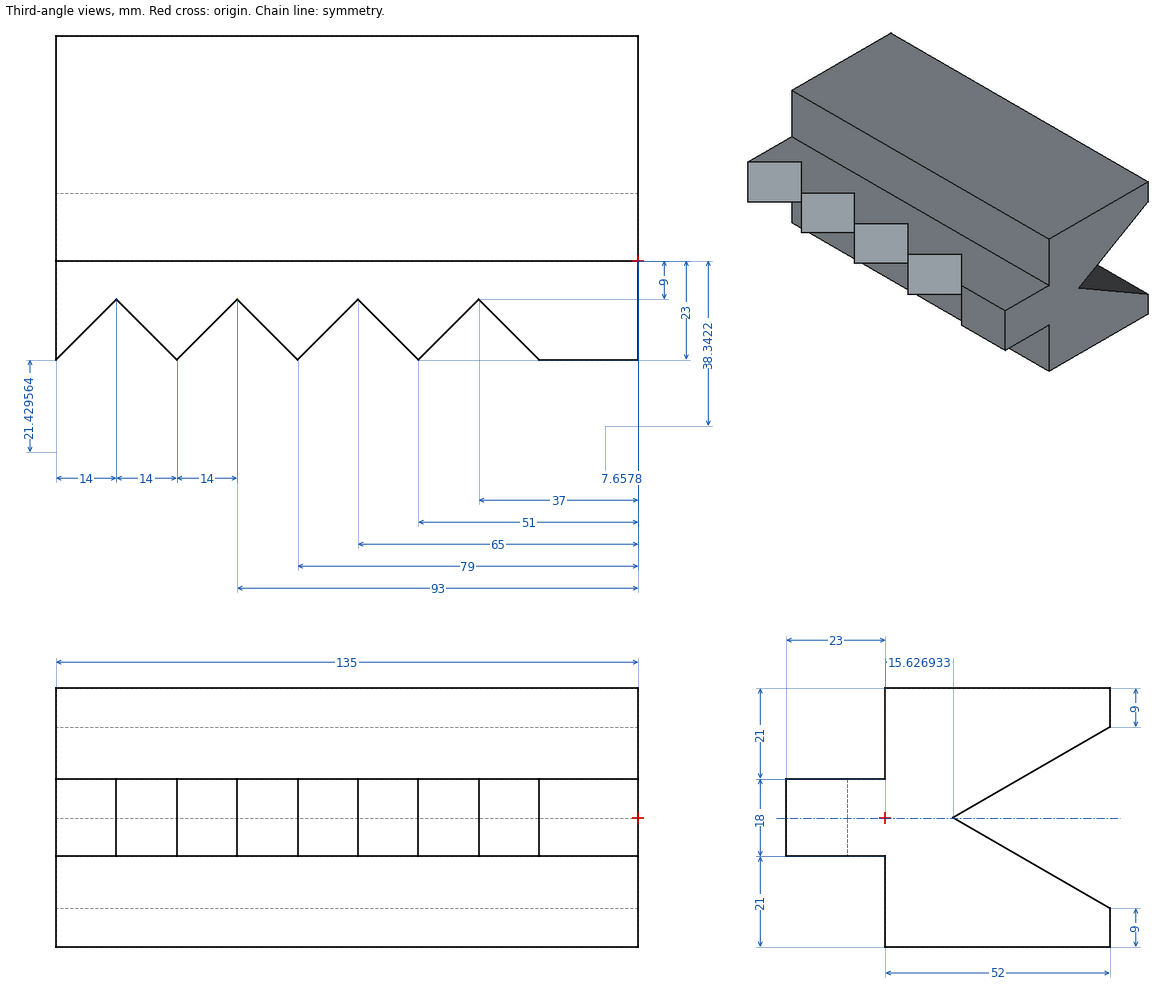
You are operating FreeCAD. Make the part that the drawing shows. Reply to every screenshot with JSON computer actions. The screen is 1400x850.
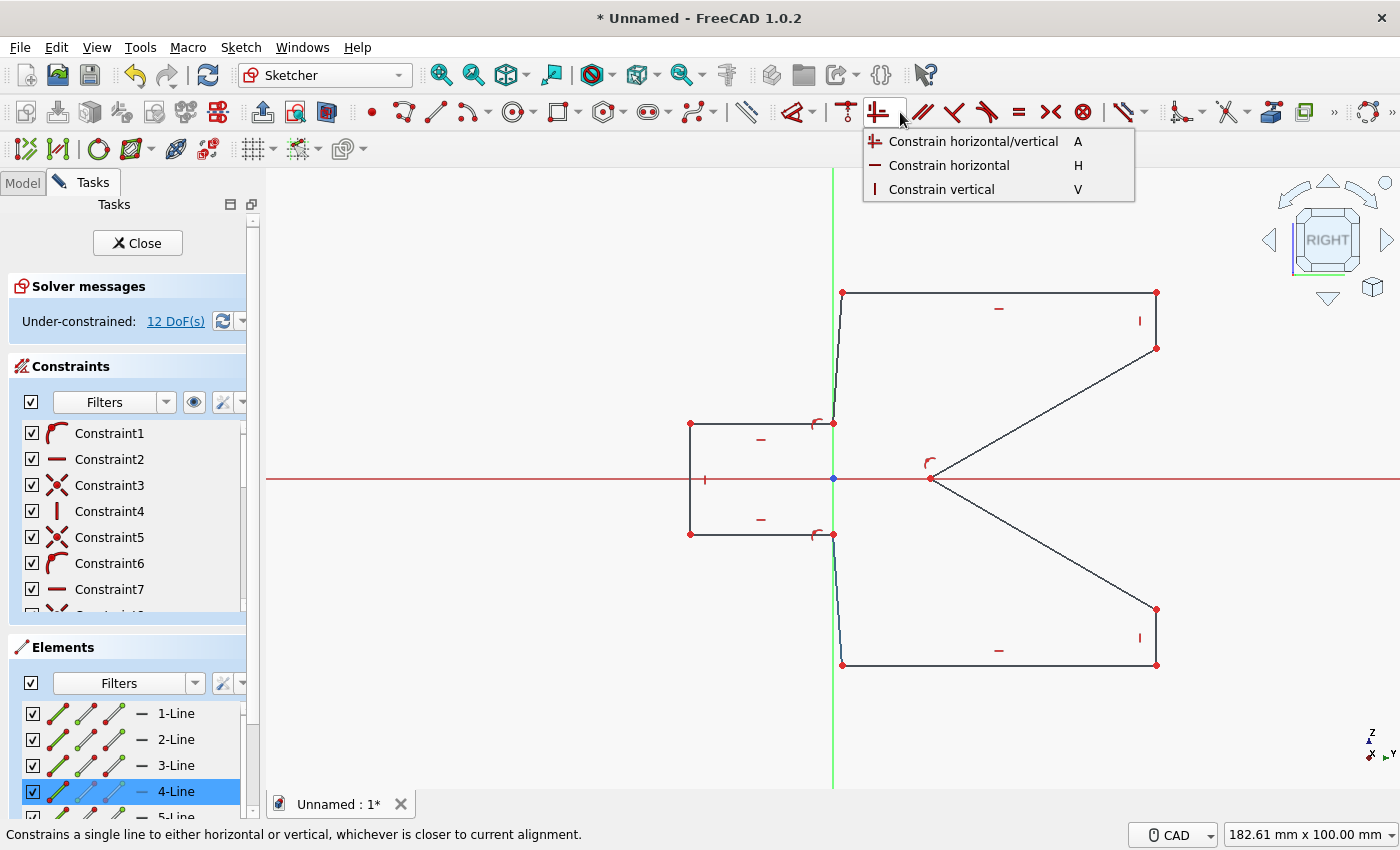
{"action": "left_click", "coordinate": [999, 189]}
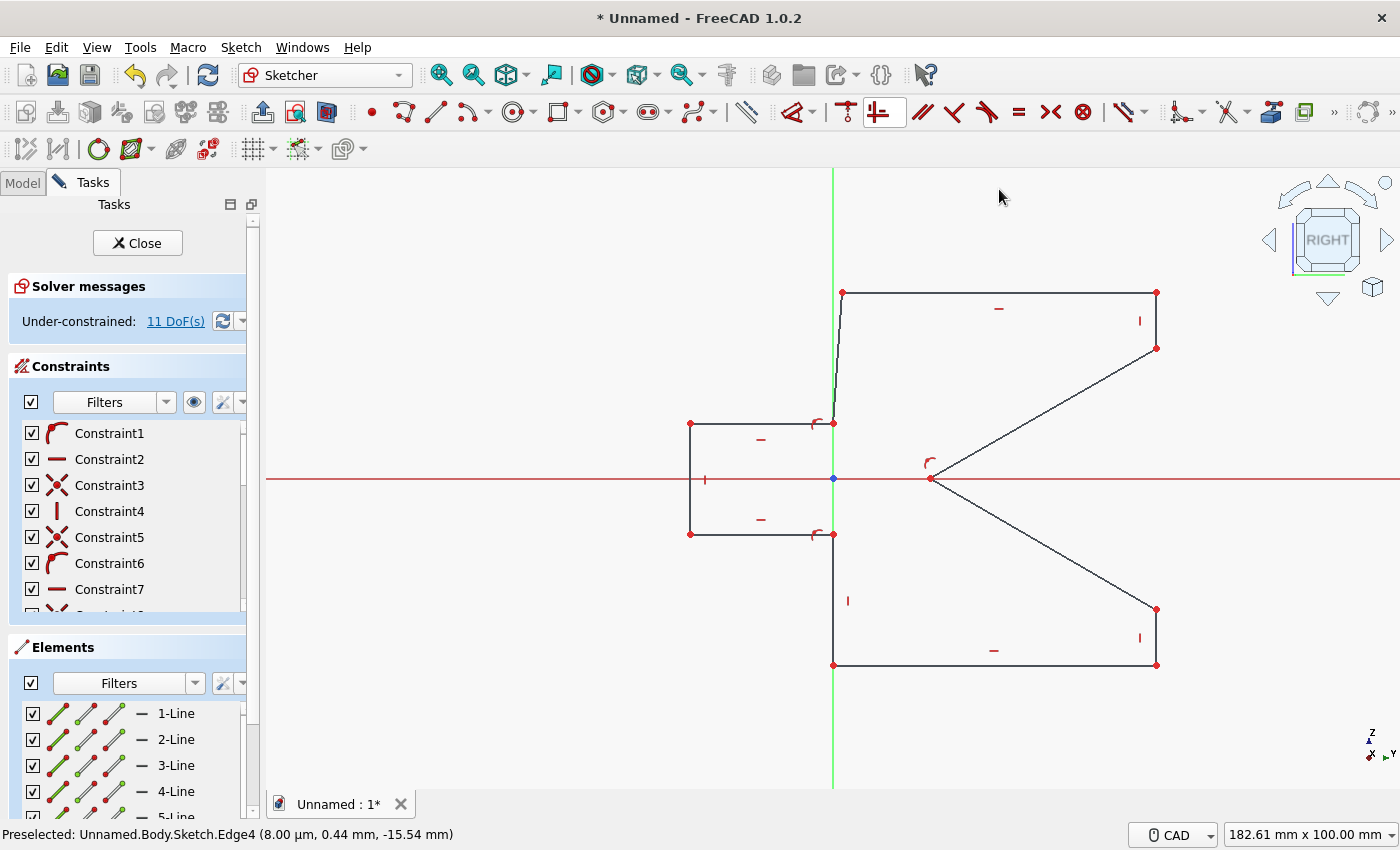
{"action": "left_click", "coordinate": [836, 385]}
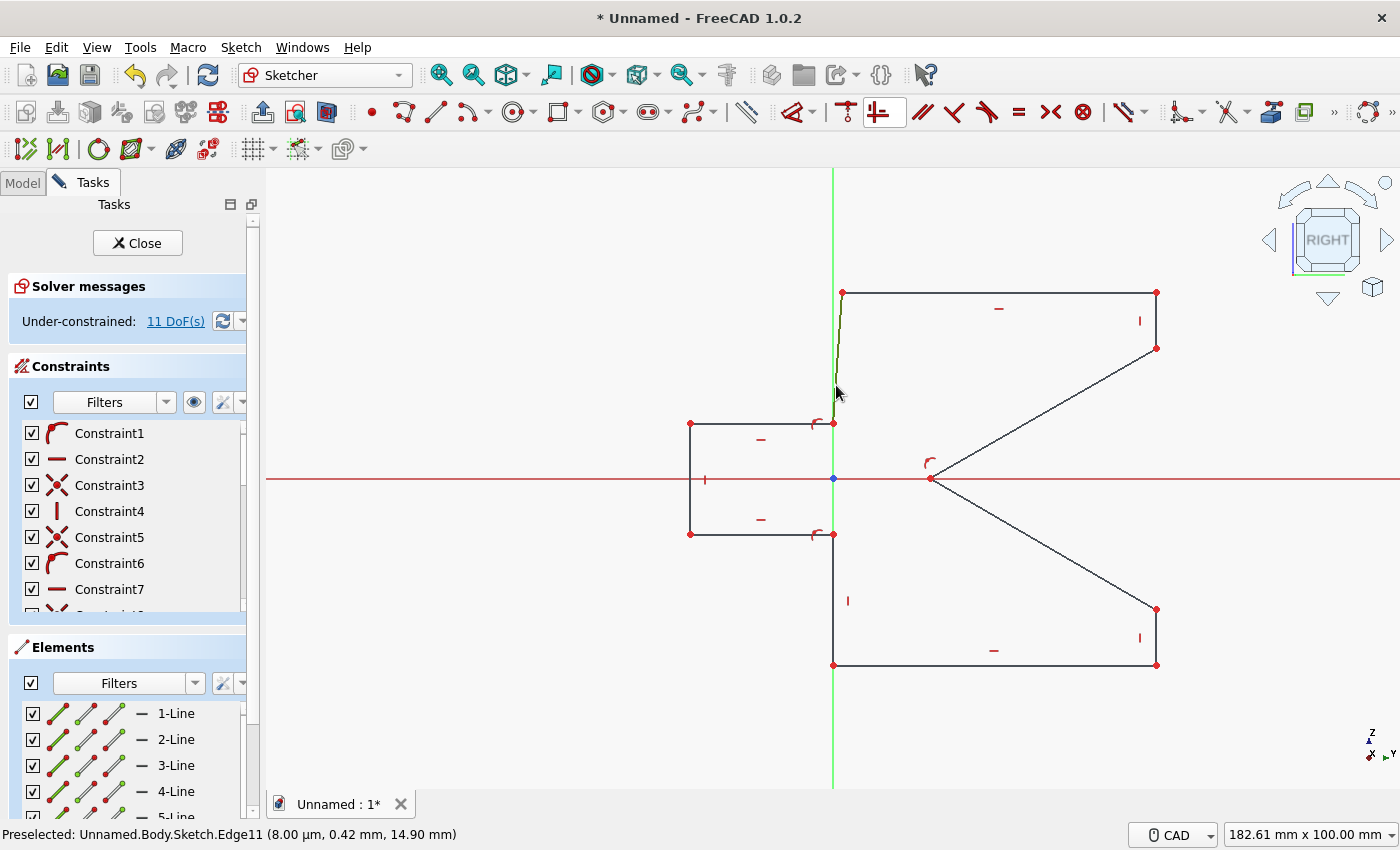
{"action": "key", "text": "v"}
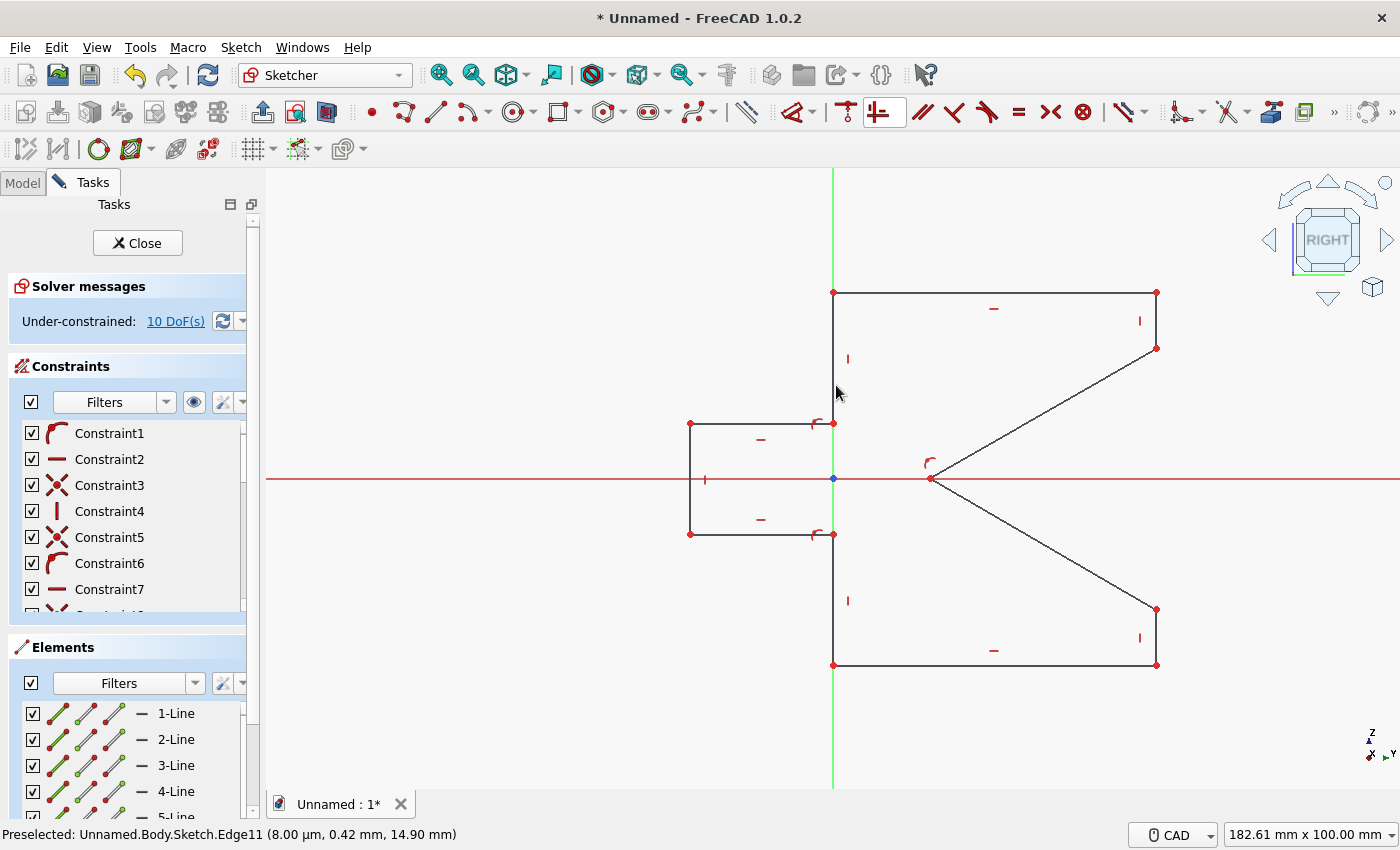
{"action": "left_click", "coordinate": [1156, 610]}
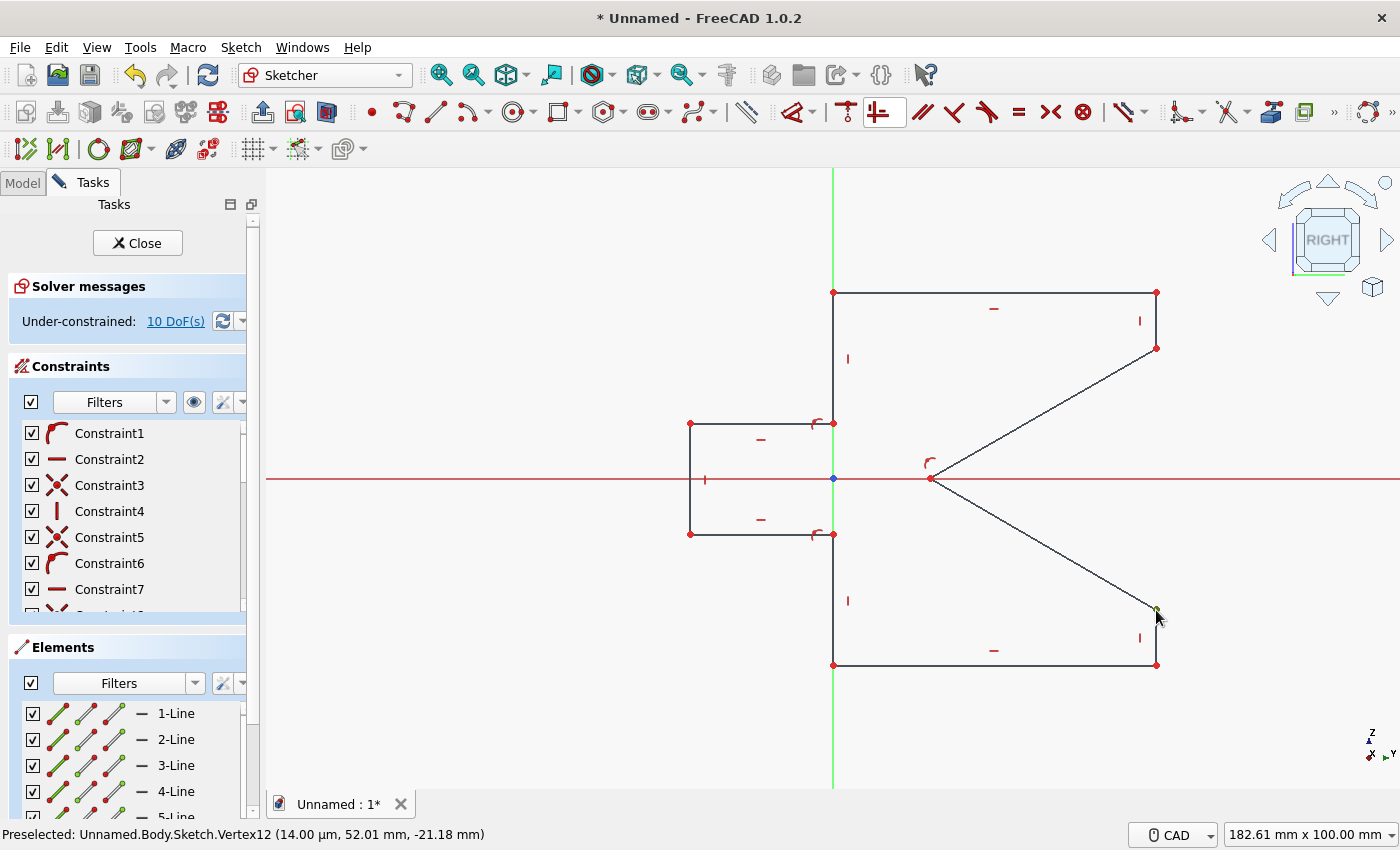
{"action": "left_click", "coordinate": [1156, 349]}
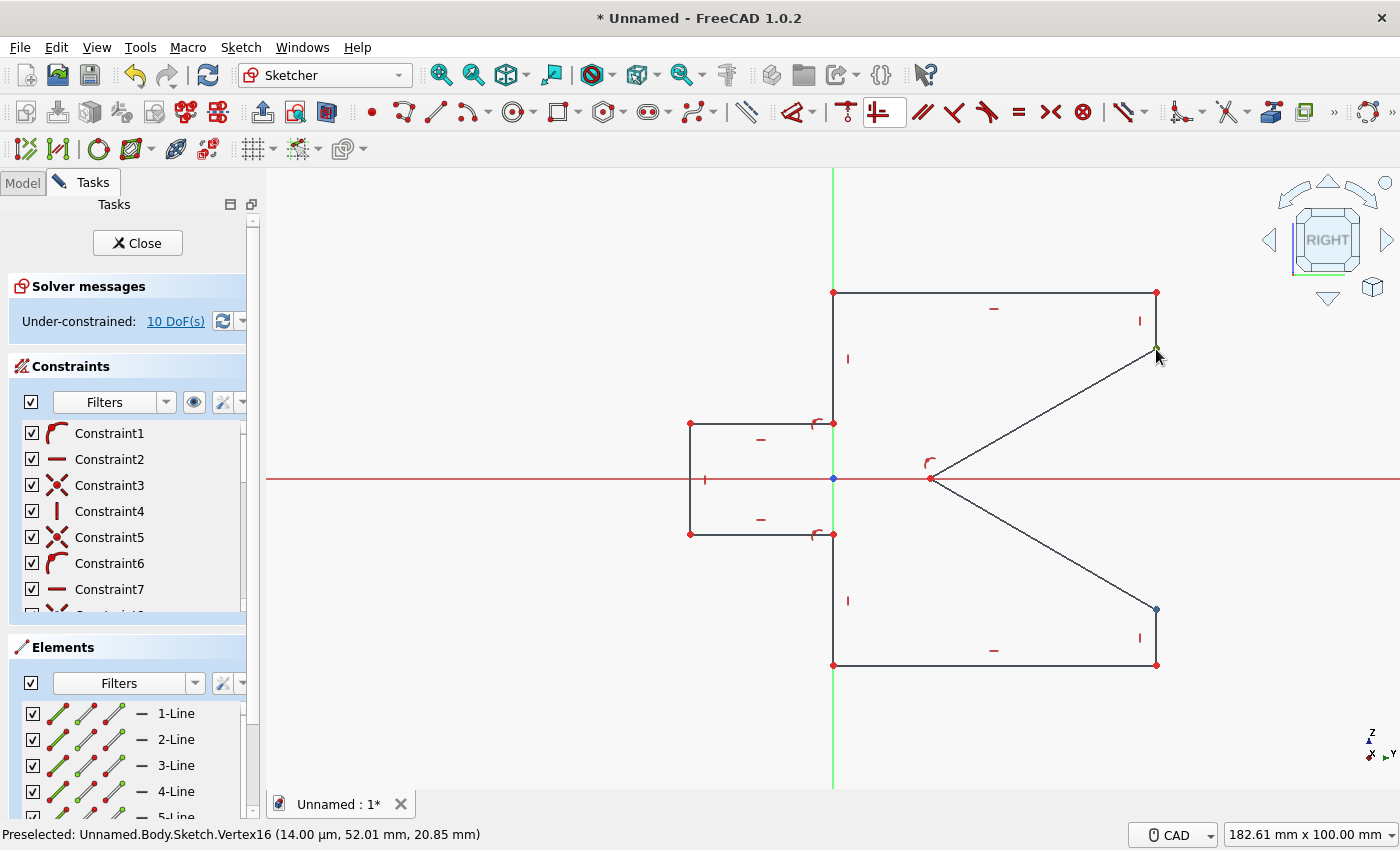
{"action": "left_click", "coordinate": [361, 478]}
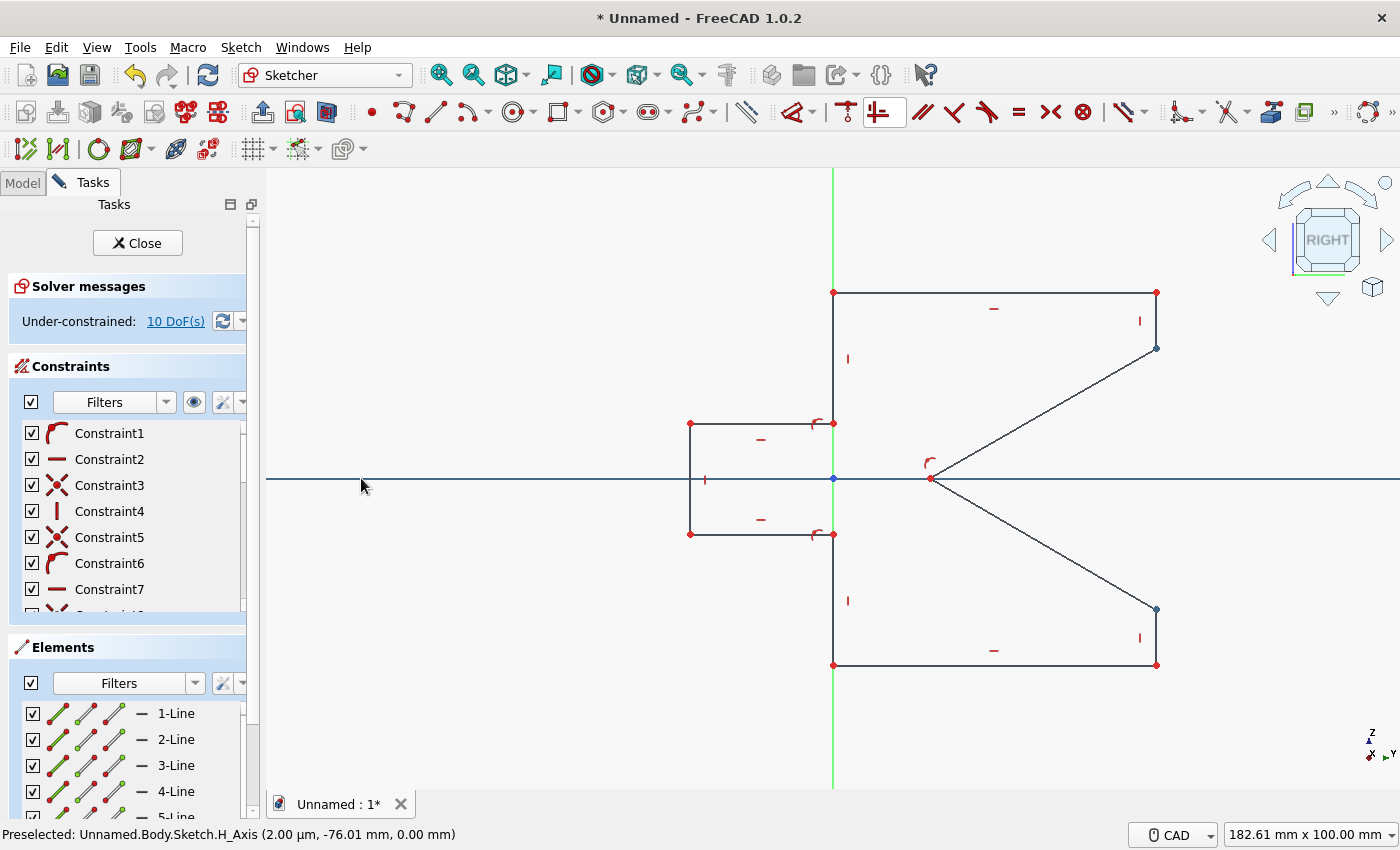
{"action": "left_click", "coordinate": [1052, 112]}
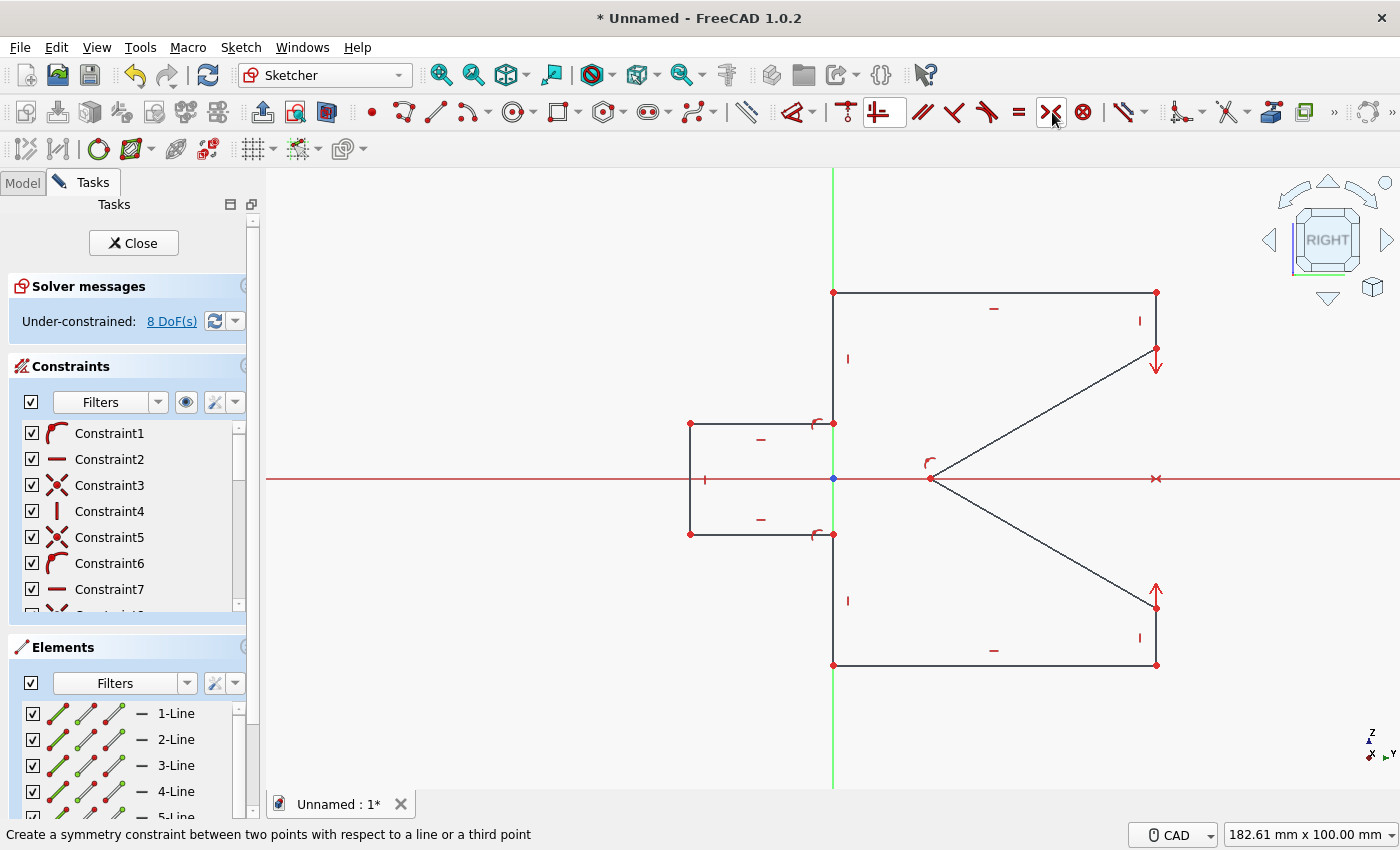
{"action": "left_click", "coordinate": [792, 112]}